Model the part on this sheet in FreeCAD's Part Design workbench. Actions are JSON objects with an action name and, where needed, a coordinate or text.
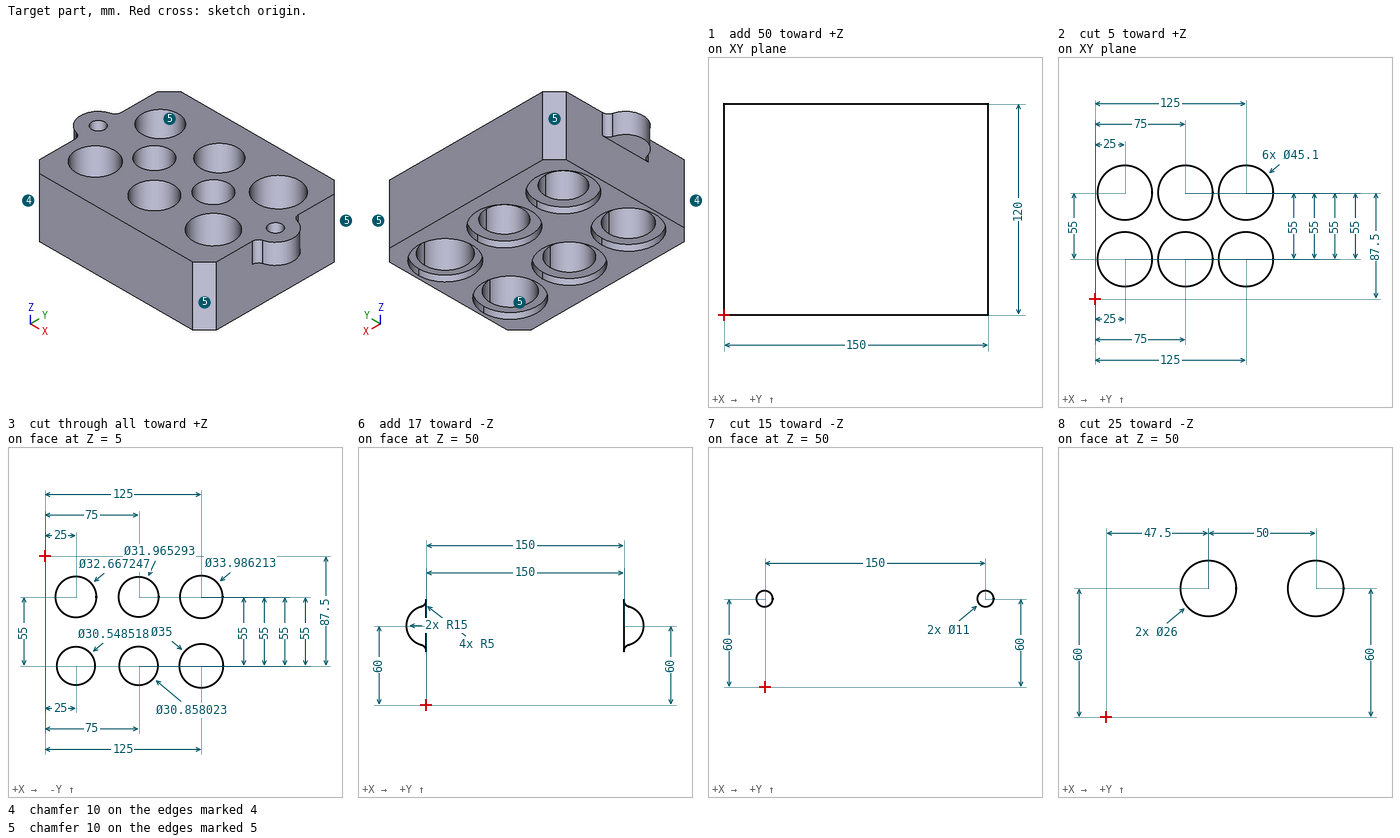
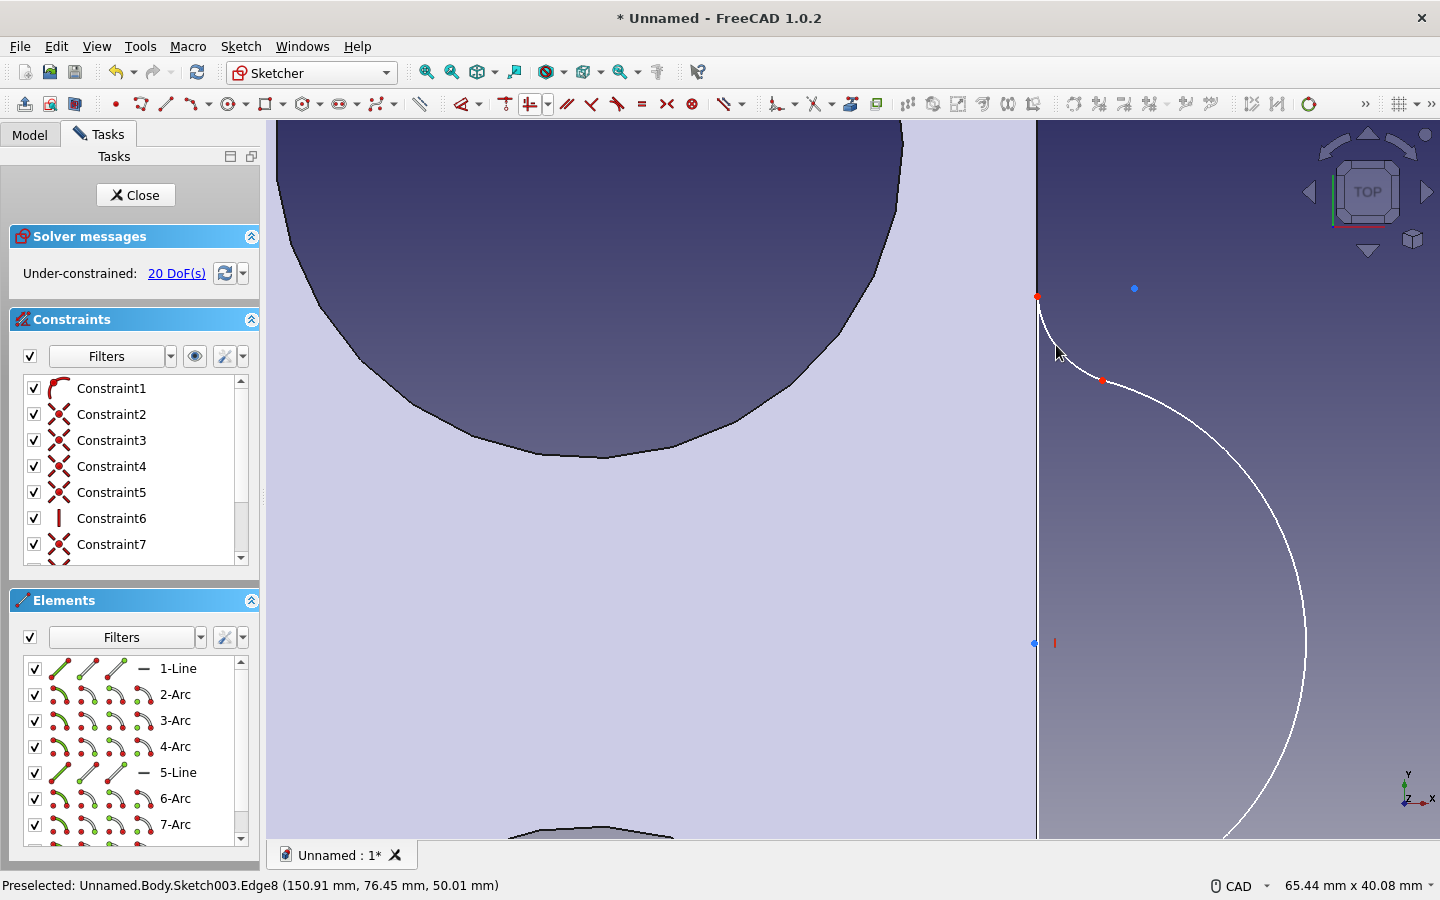
{"action": "scroll", "coordinate": [1061, 347], "scroll_direction": "down", "scroll_amount": 8}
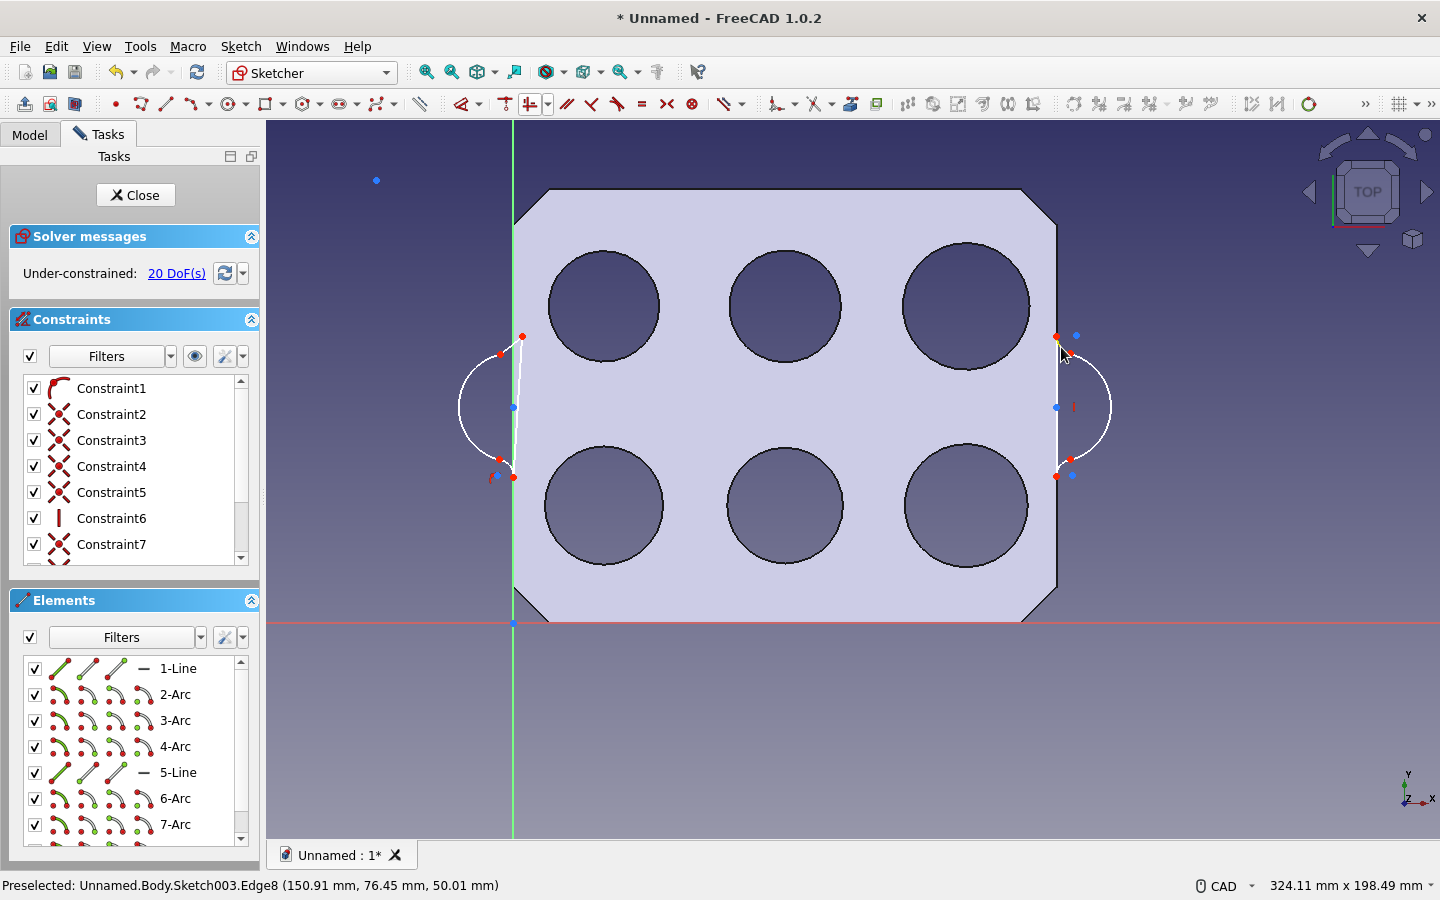
{"action": "scroll", "coordinate": [516, 435], "scroll_direction": "up", "scroll_amount": 9}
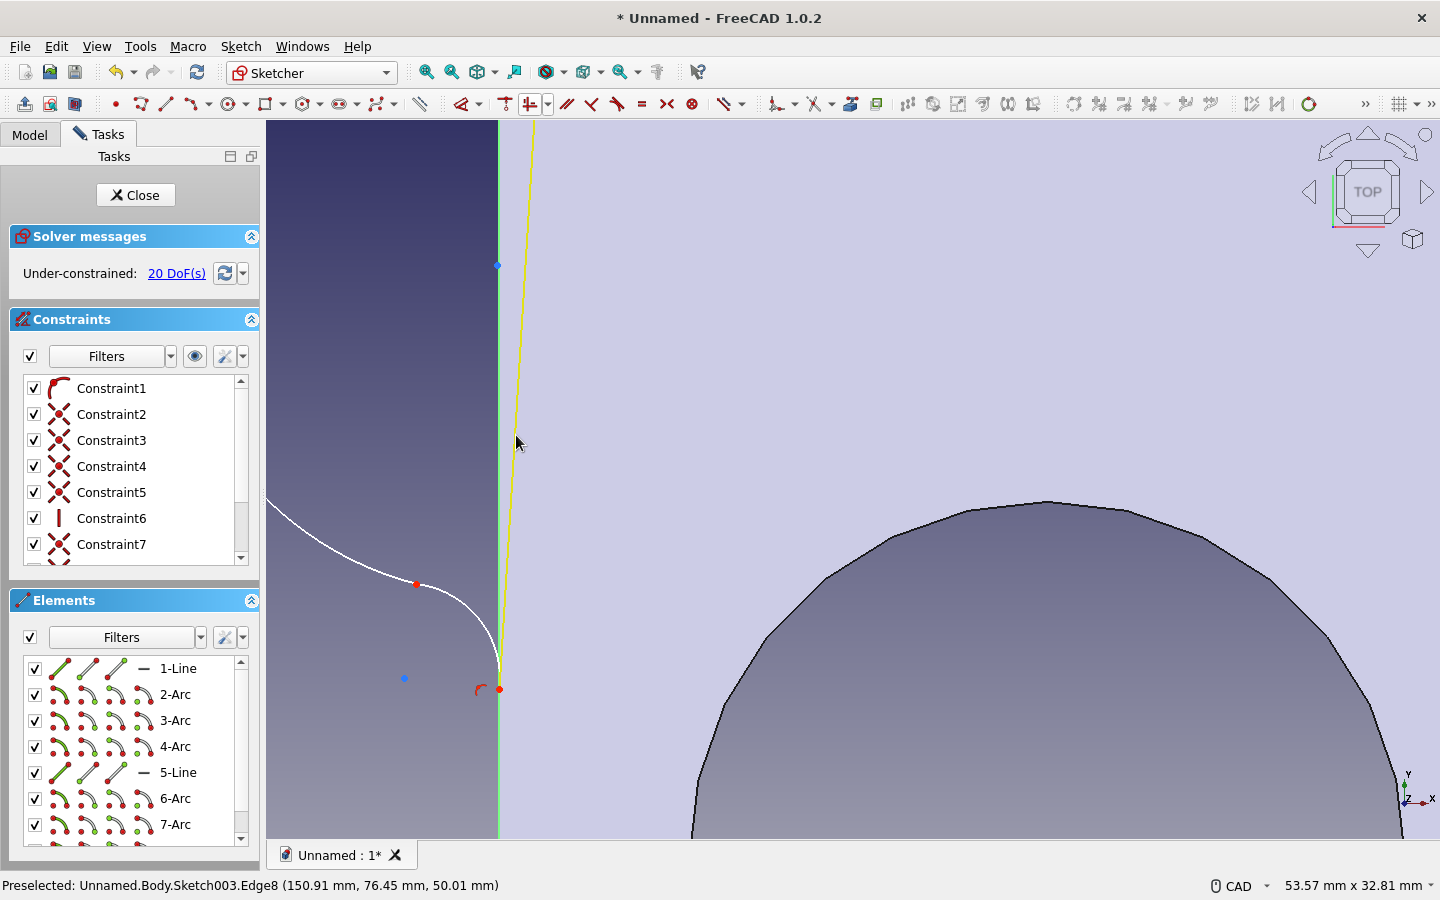
{"action": "left_click", "coordinate": [515, 434]}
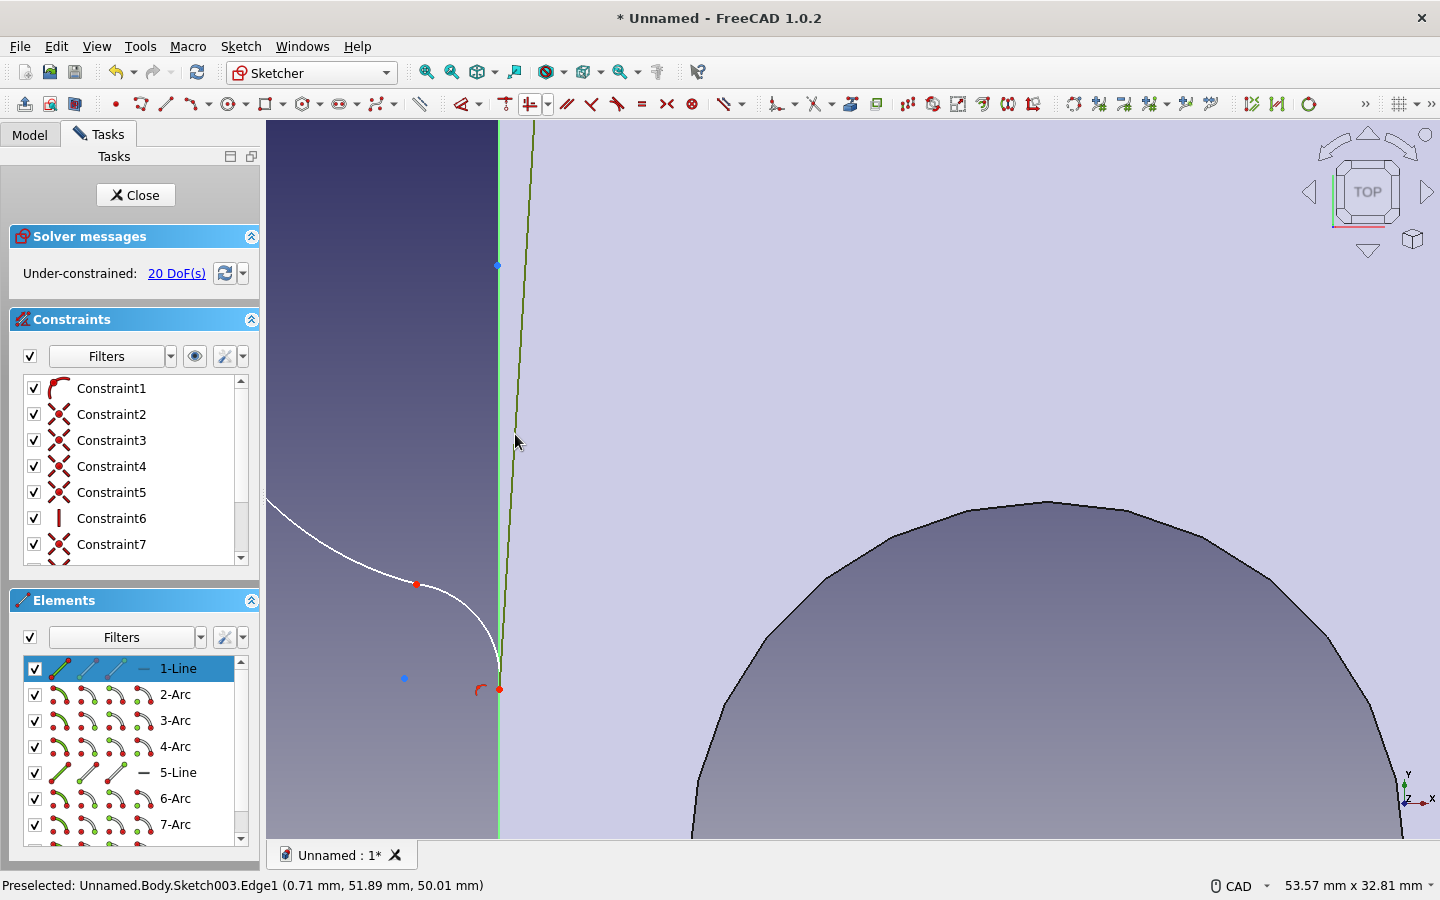
{"action": "scroll", "coordinate": [515, 435], "scroll_direction": "down", "scroll_amount": 9}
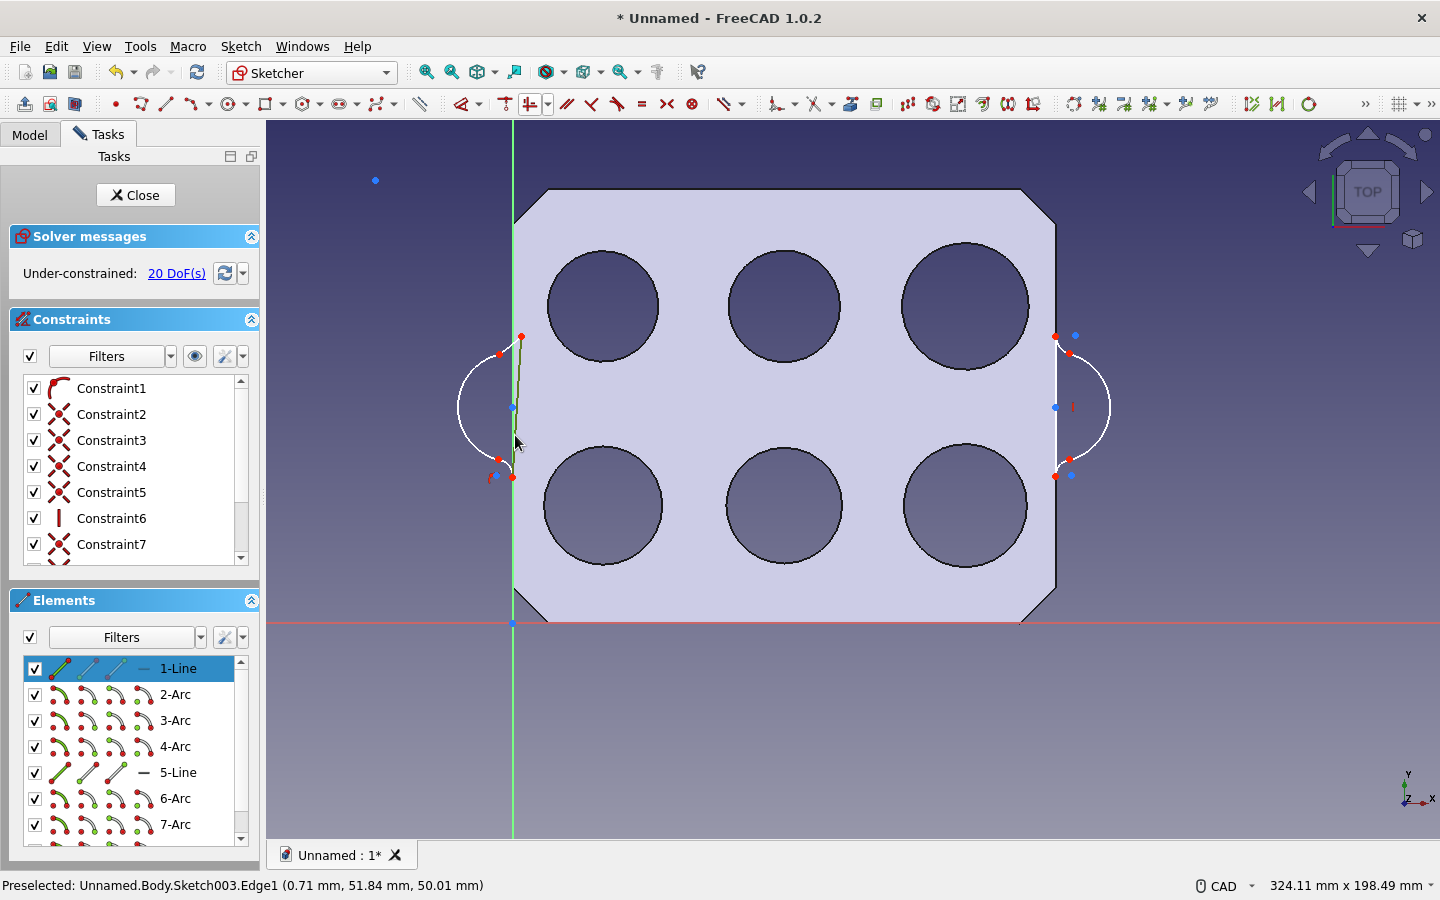
{"action": "scroll", "coordinate": [506, 349], "scroll_direction": "up", "scroll_amount": 4}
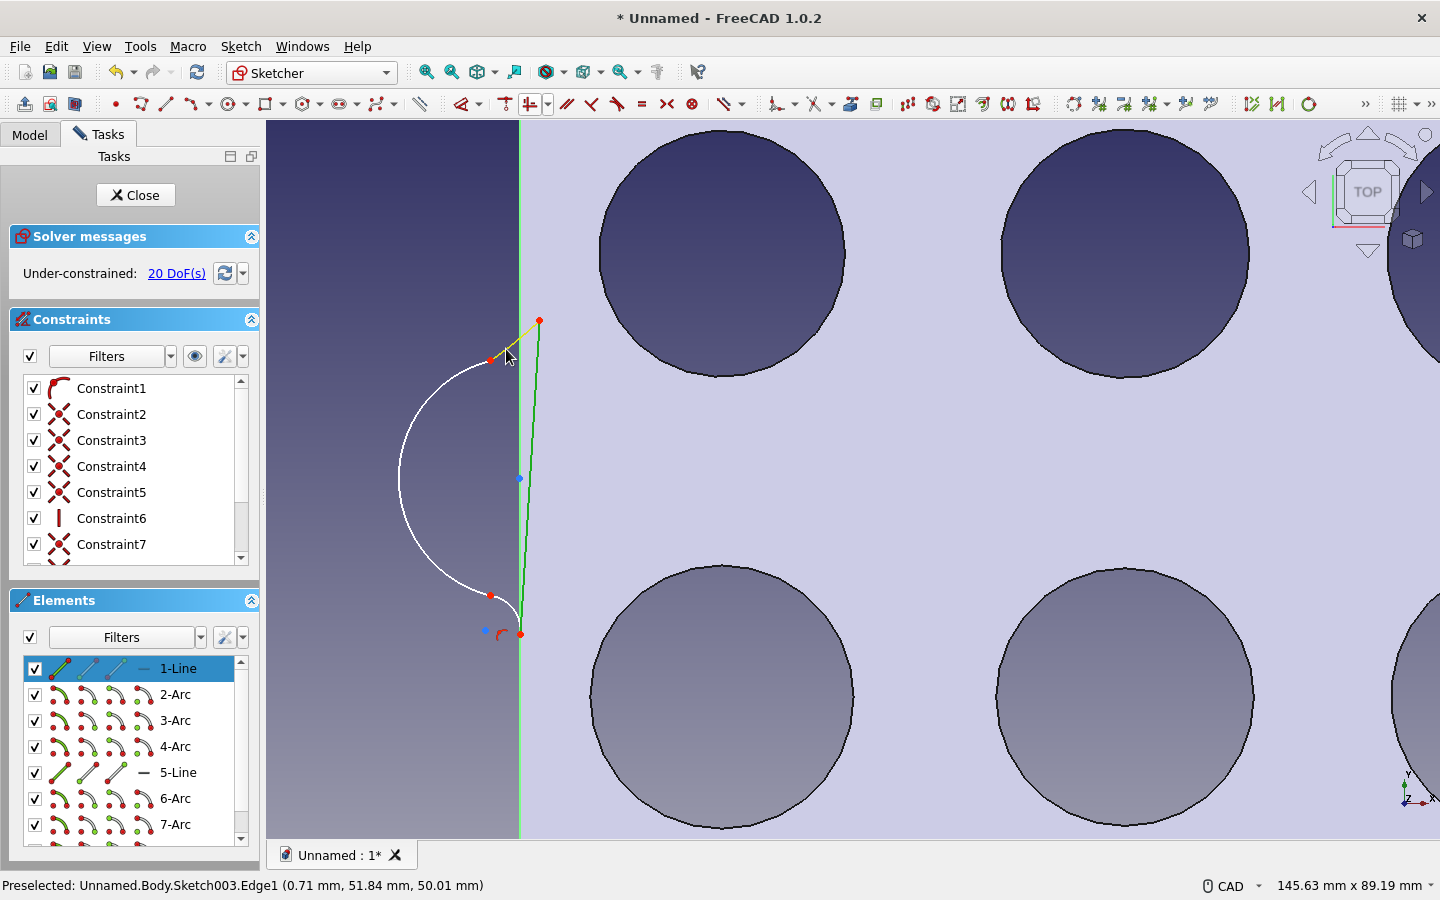
{"action": "left_click", "coordinate": [506, 349]}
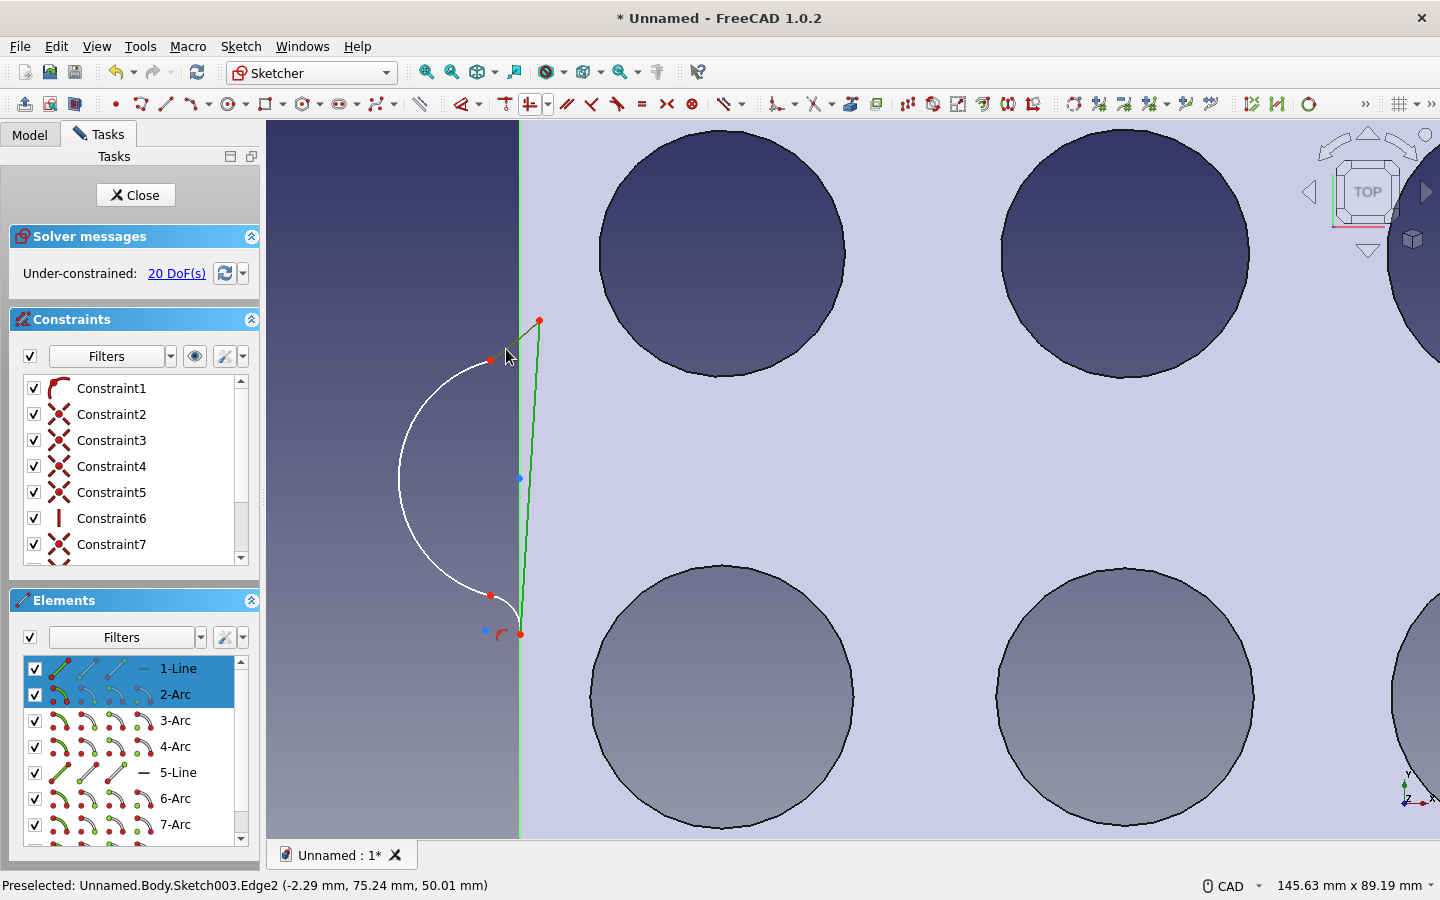
{"action": "left_click", "coordinate": [617, 104]}